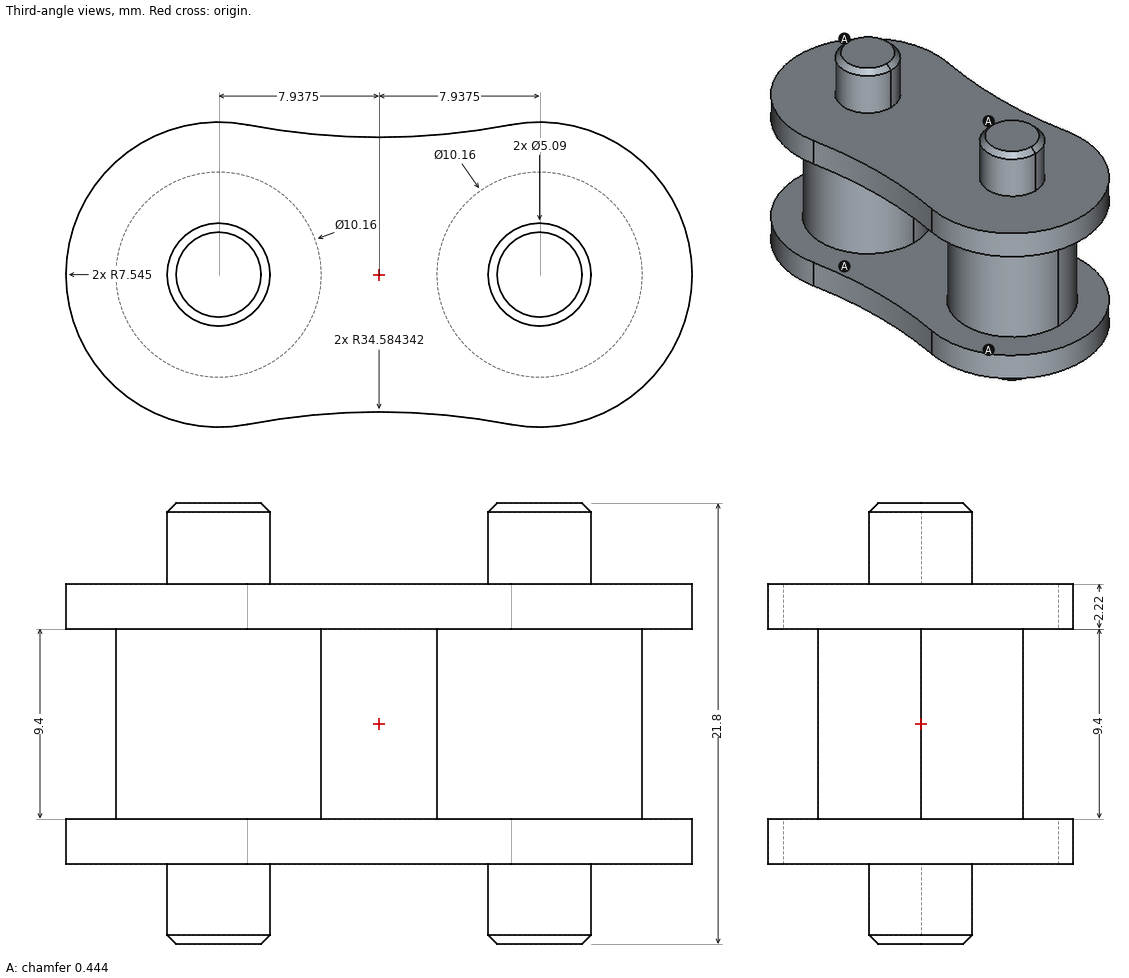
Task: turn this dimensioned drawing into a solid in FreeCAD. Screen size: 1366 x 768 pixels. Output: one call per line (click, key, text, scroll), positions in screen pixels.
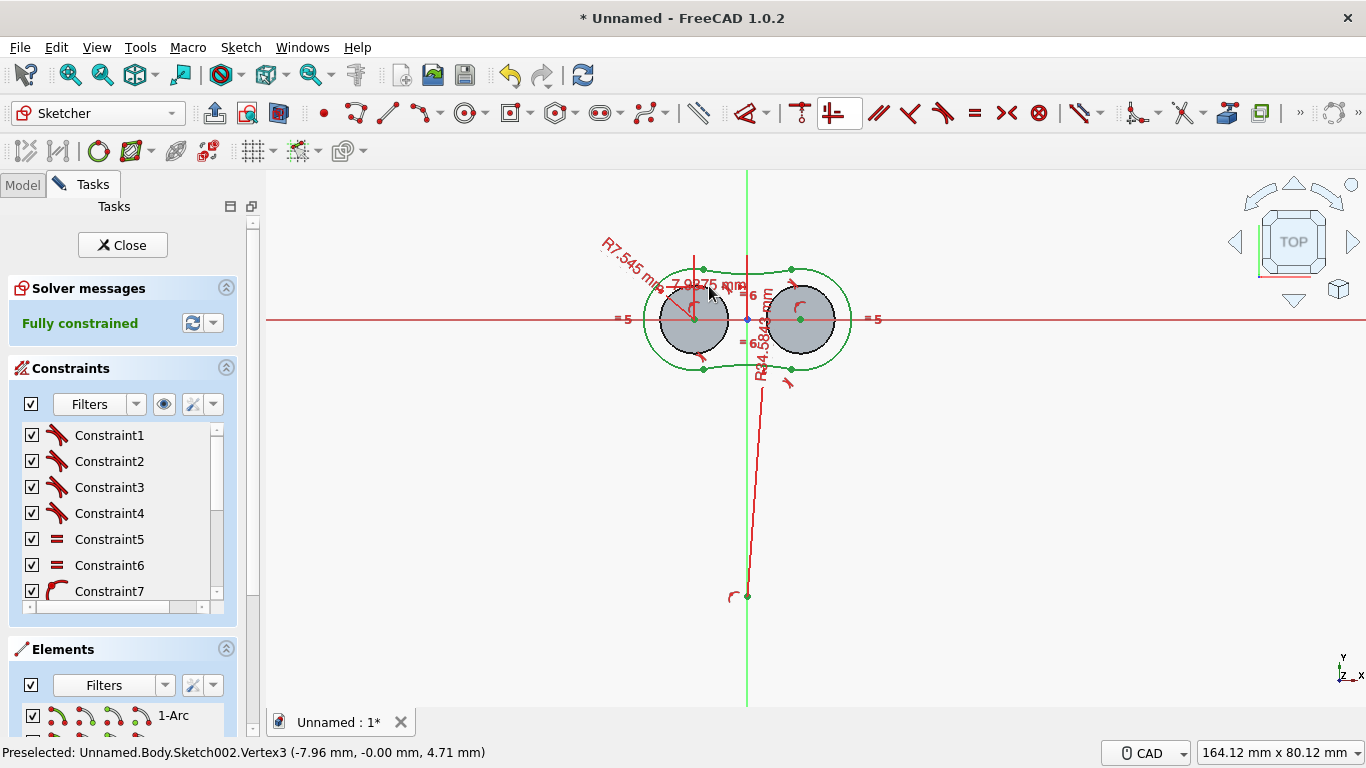
click(123, 245)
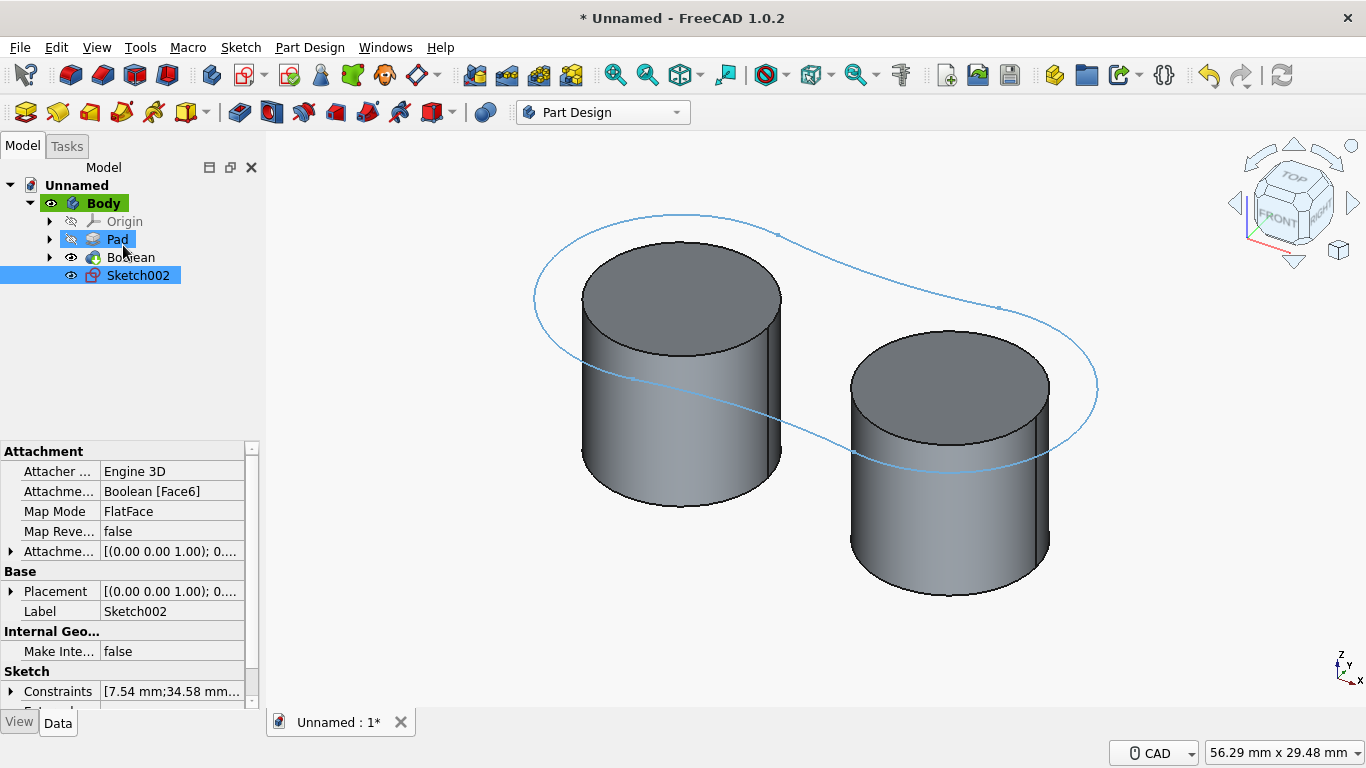
click(26, 112)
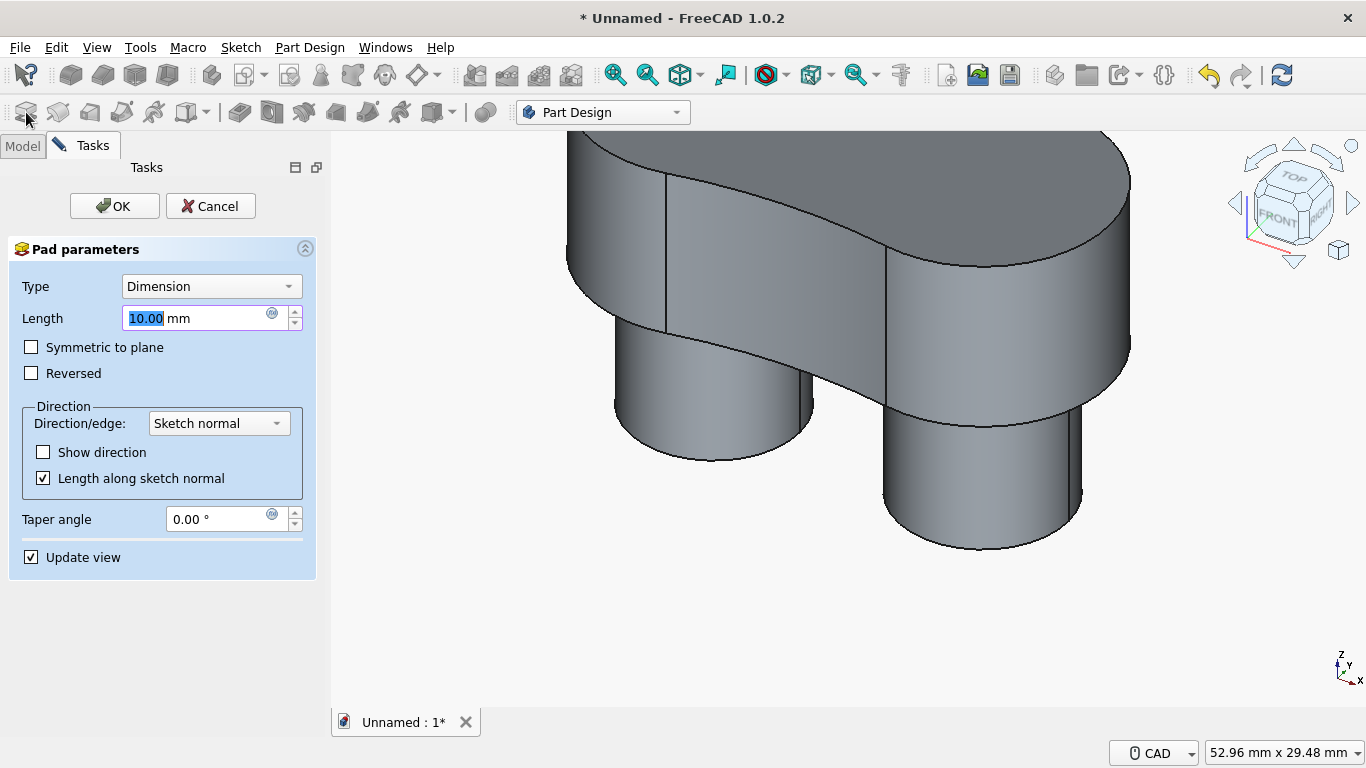
text(2.22)
key(Tab)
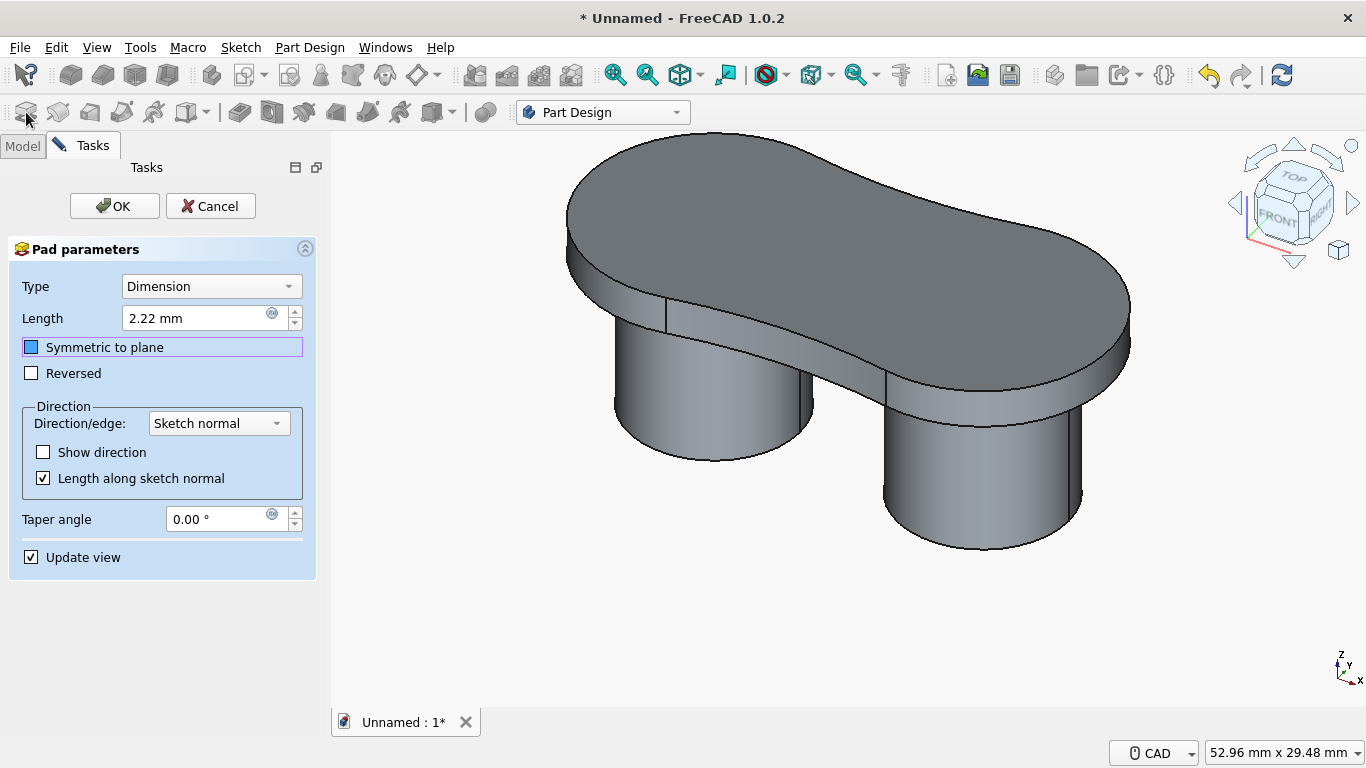
click(115, 206)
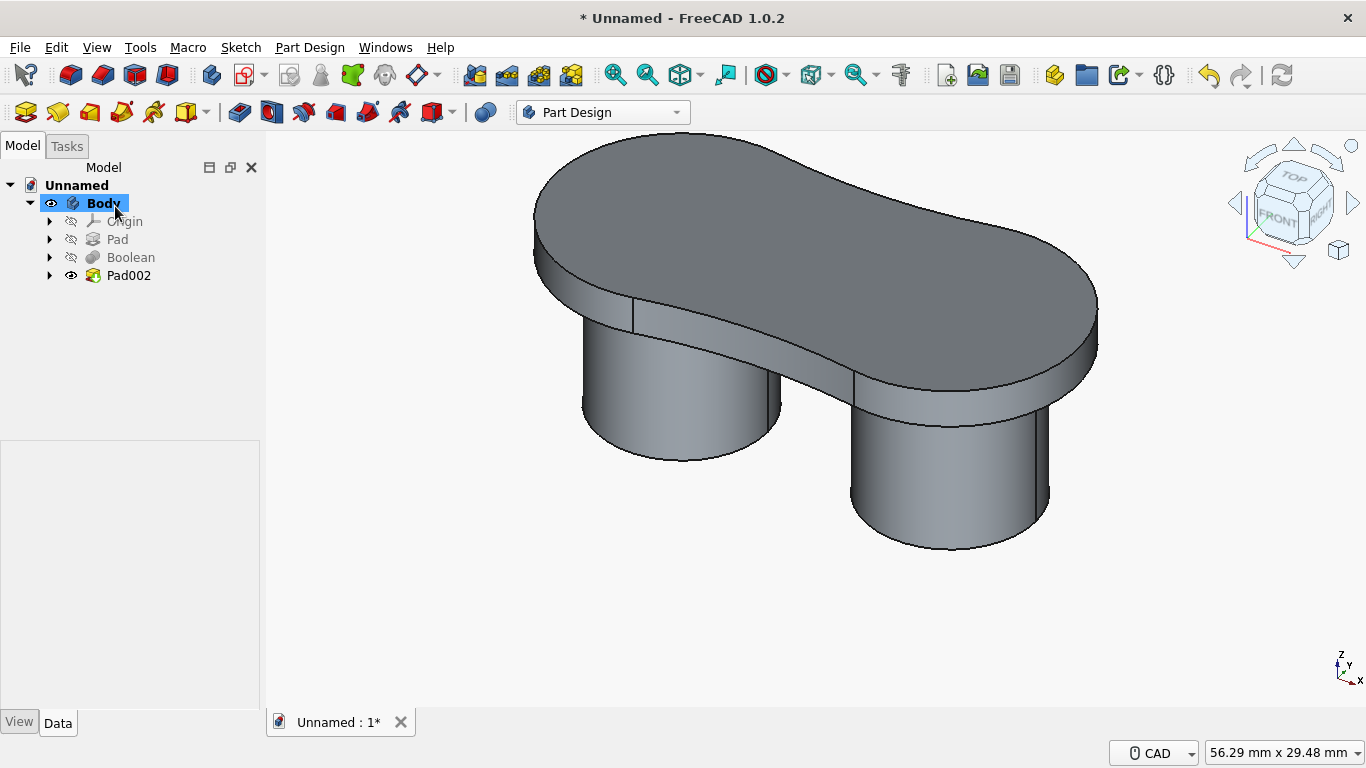
key(v)
key(f)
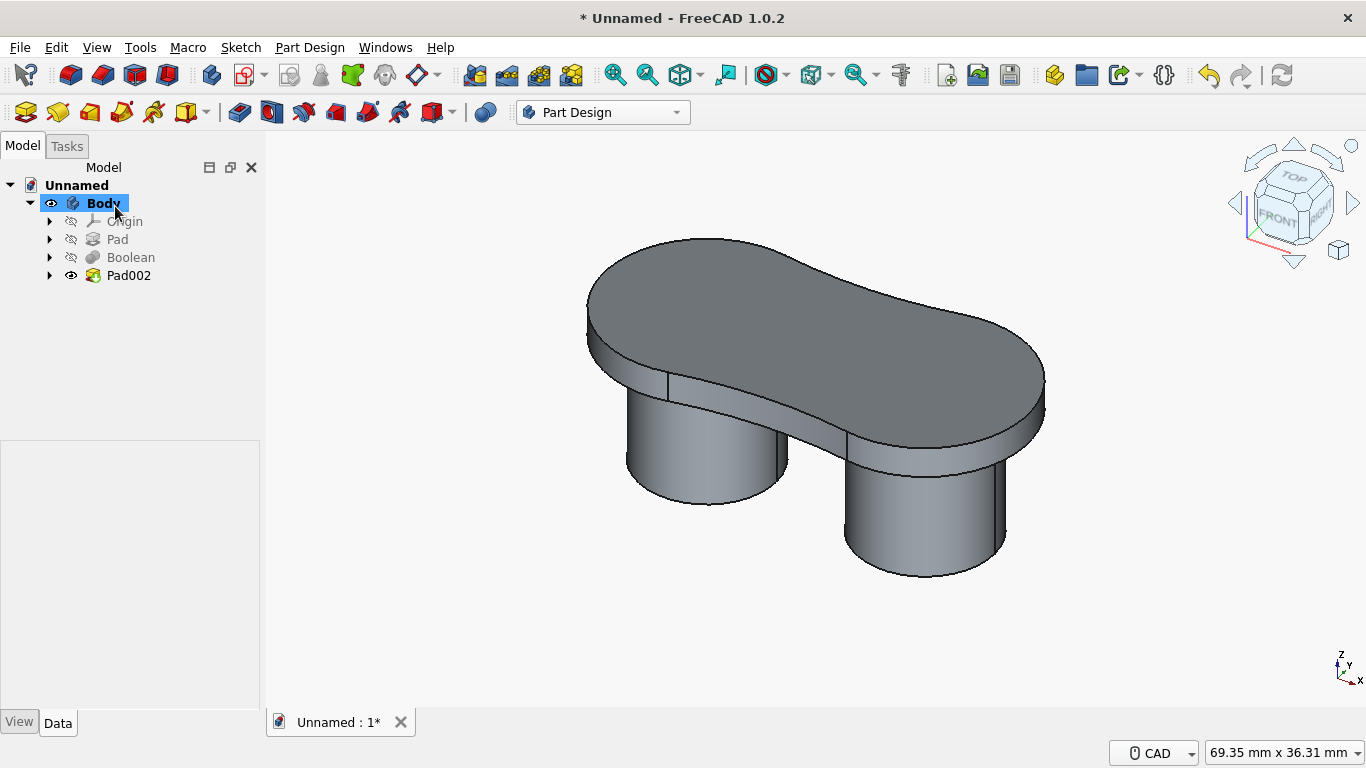
click(116, 275)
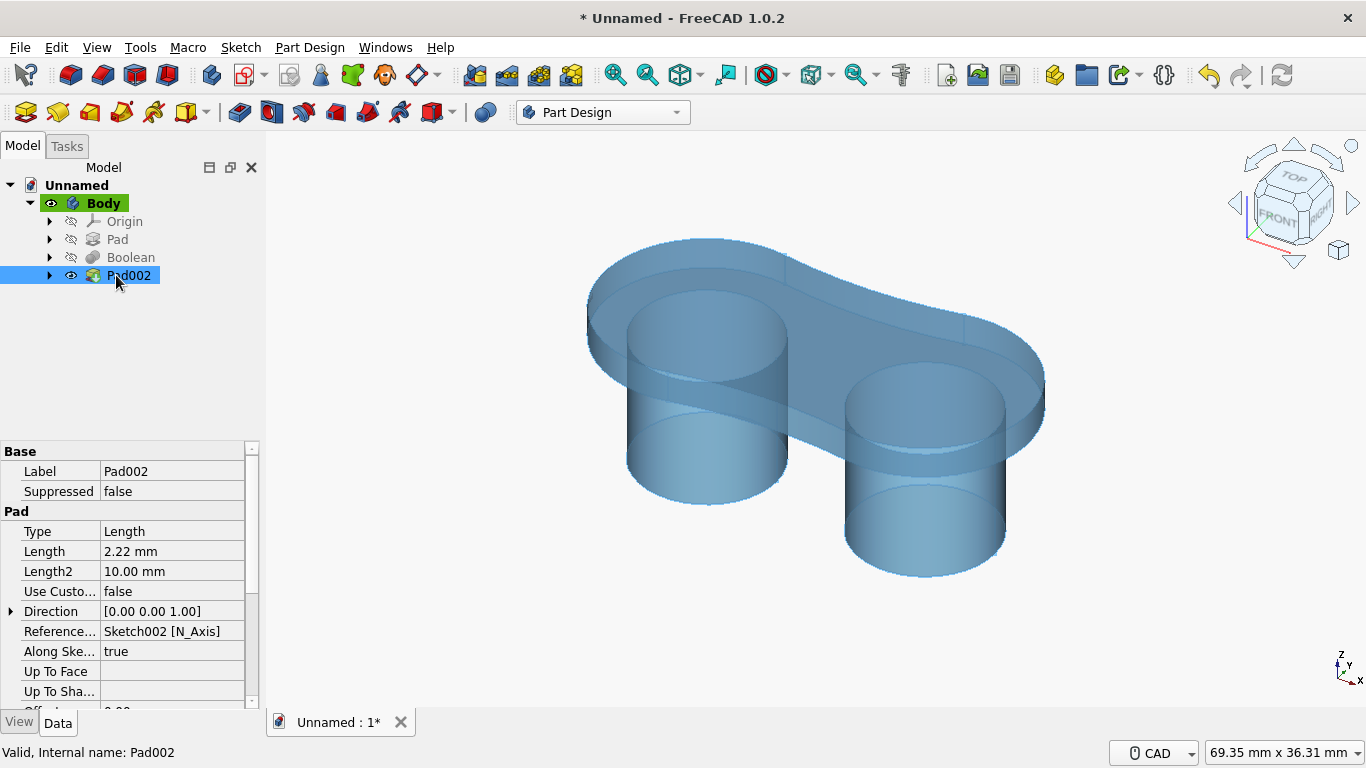
click(476, 76)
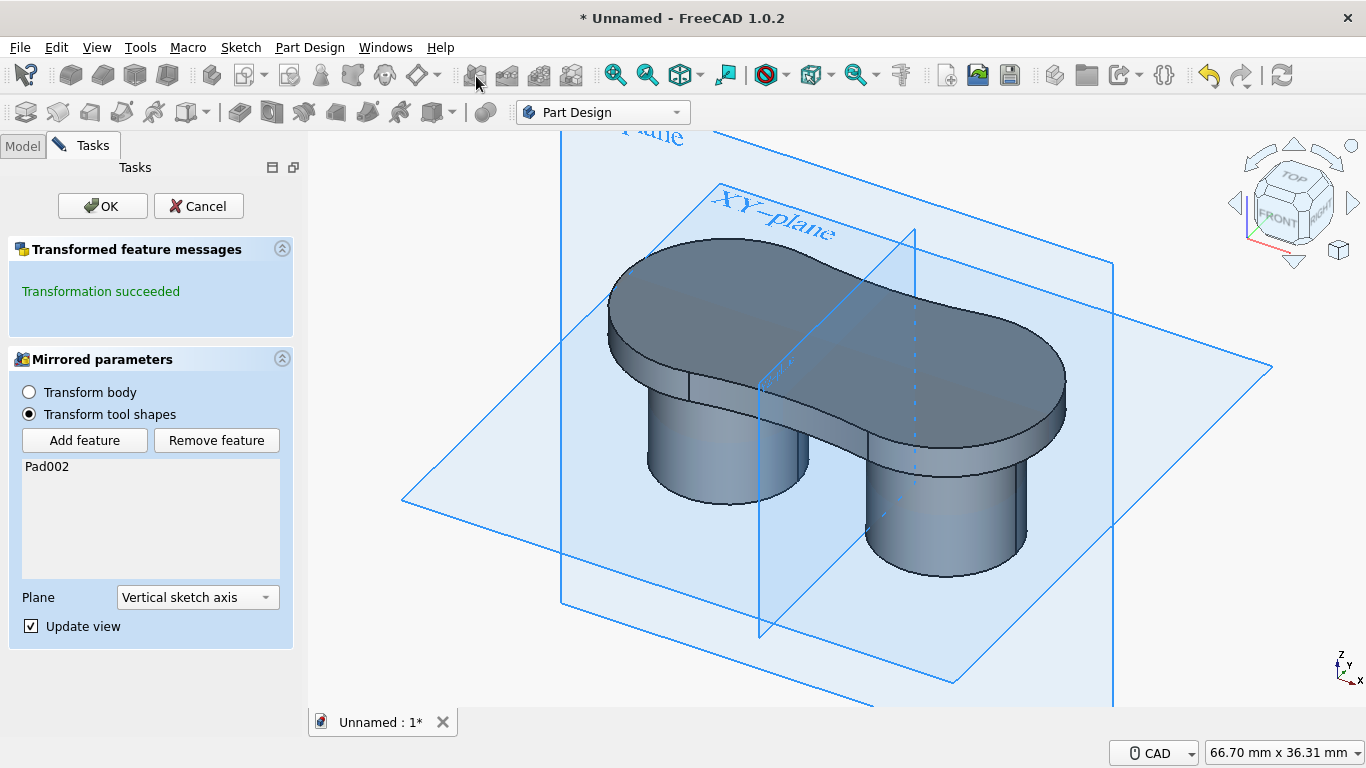
click(198, 598)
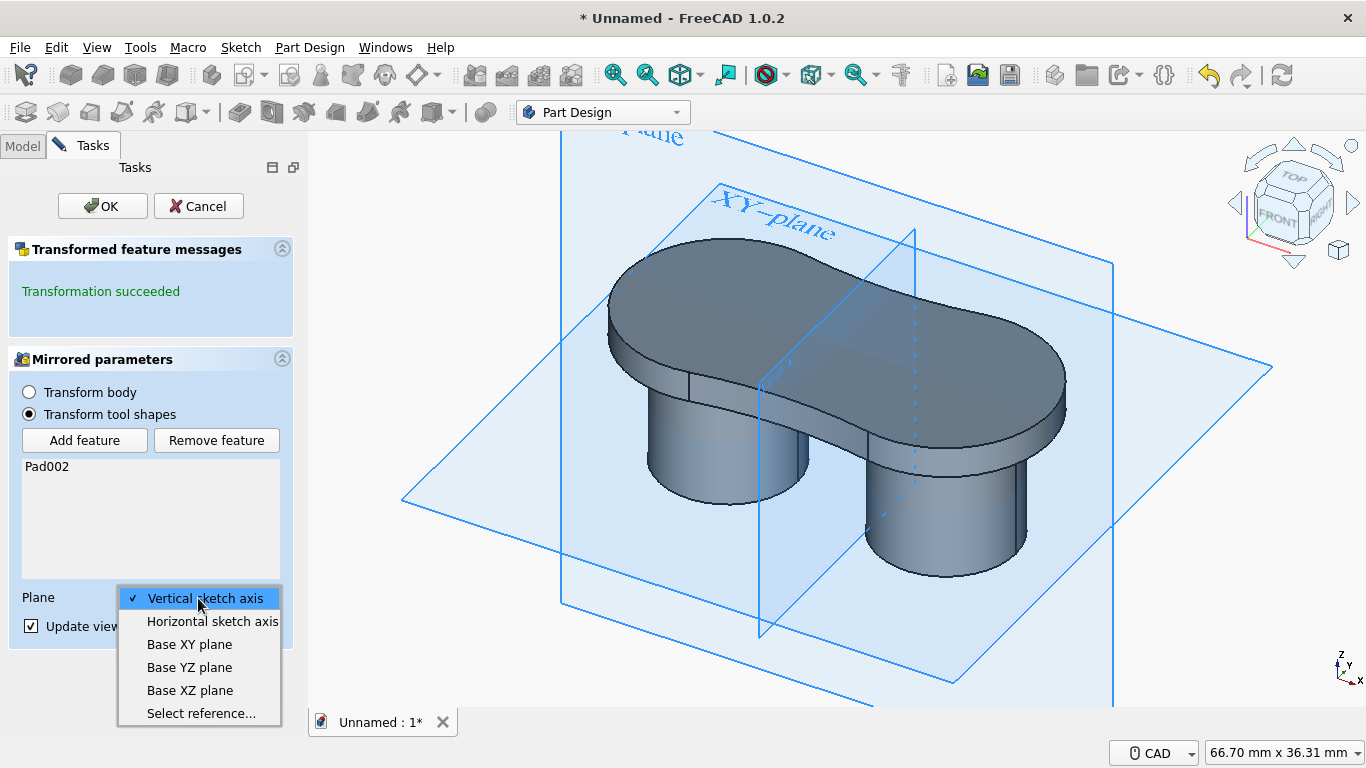
click(198, 644)